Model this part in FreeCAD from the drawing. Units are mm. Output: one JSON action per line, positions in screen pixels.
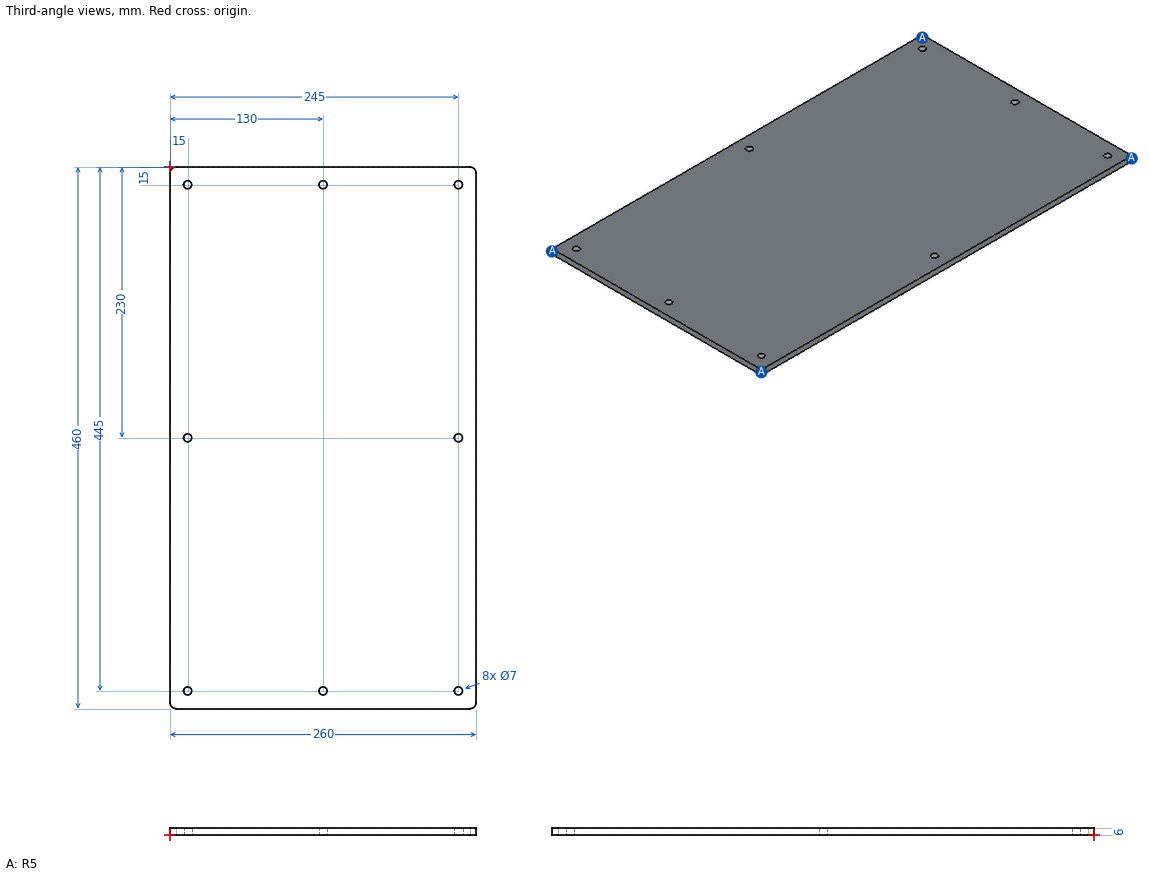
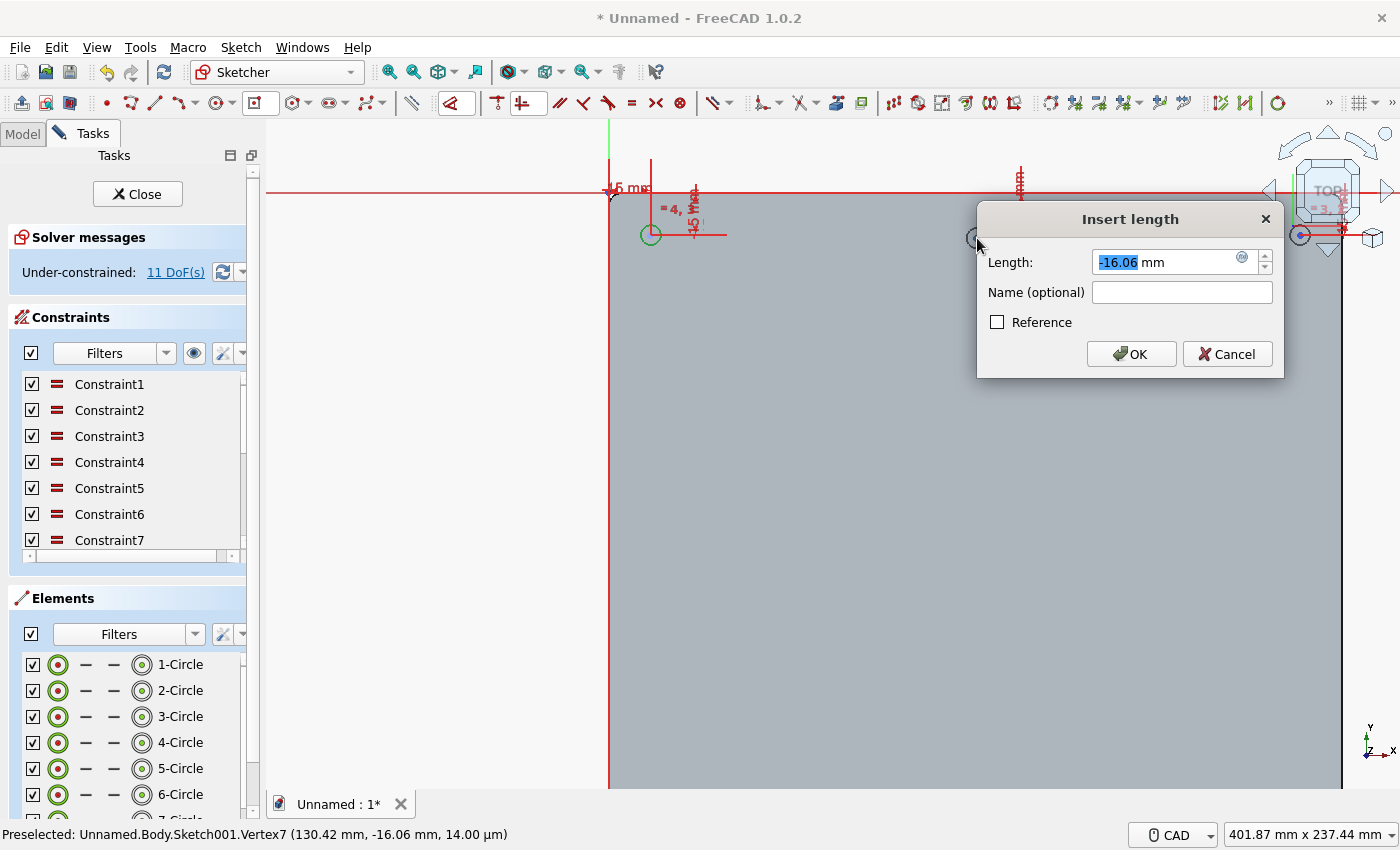
{"action": "type", "text": "-15"}
{"action": "key", "text": "Return"}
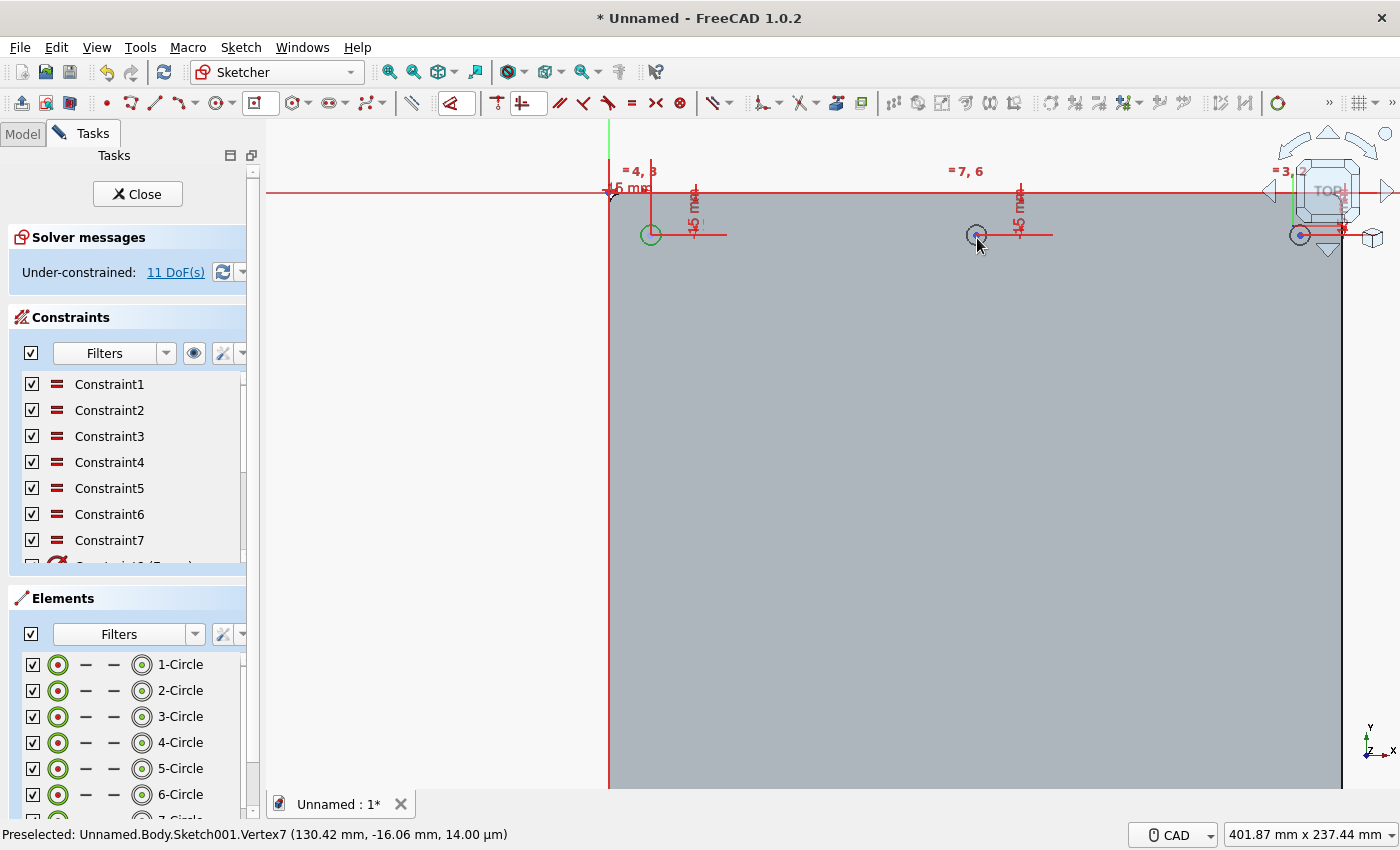
{"action": "scroll", "coordinate": [651, 238], "scroll_direction": "down", "scroll_amount": 5}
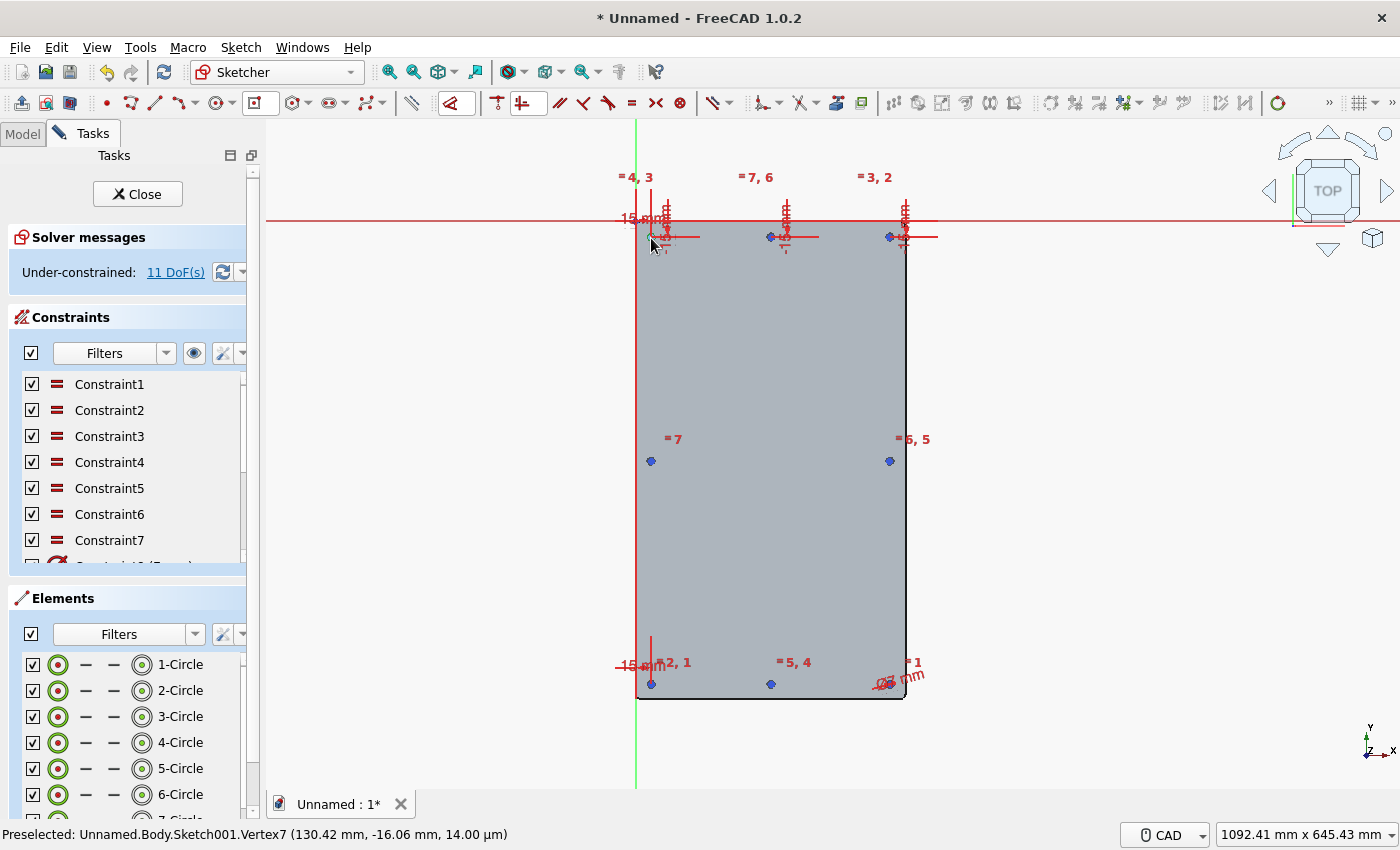
{"action": "scroll", "coordinate": [651, 461], "scroll_direction": "up", "scroll_amount": 5}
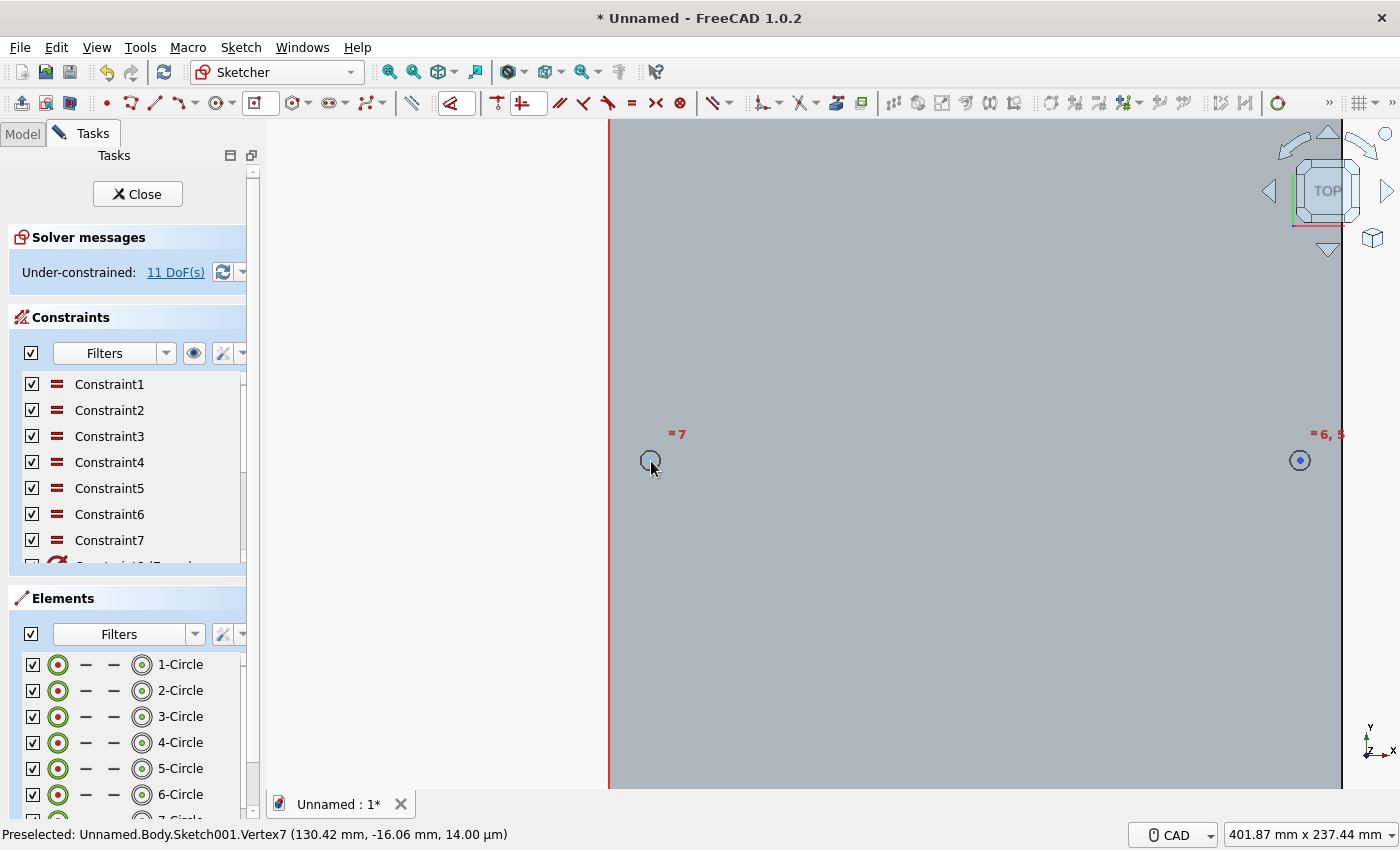
{"action": "left_click", "coordinate": [650, 461]}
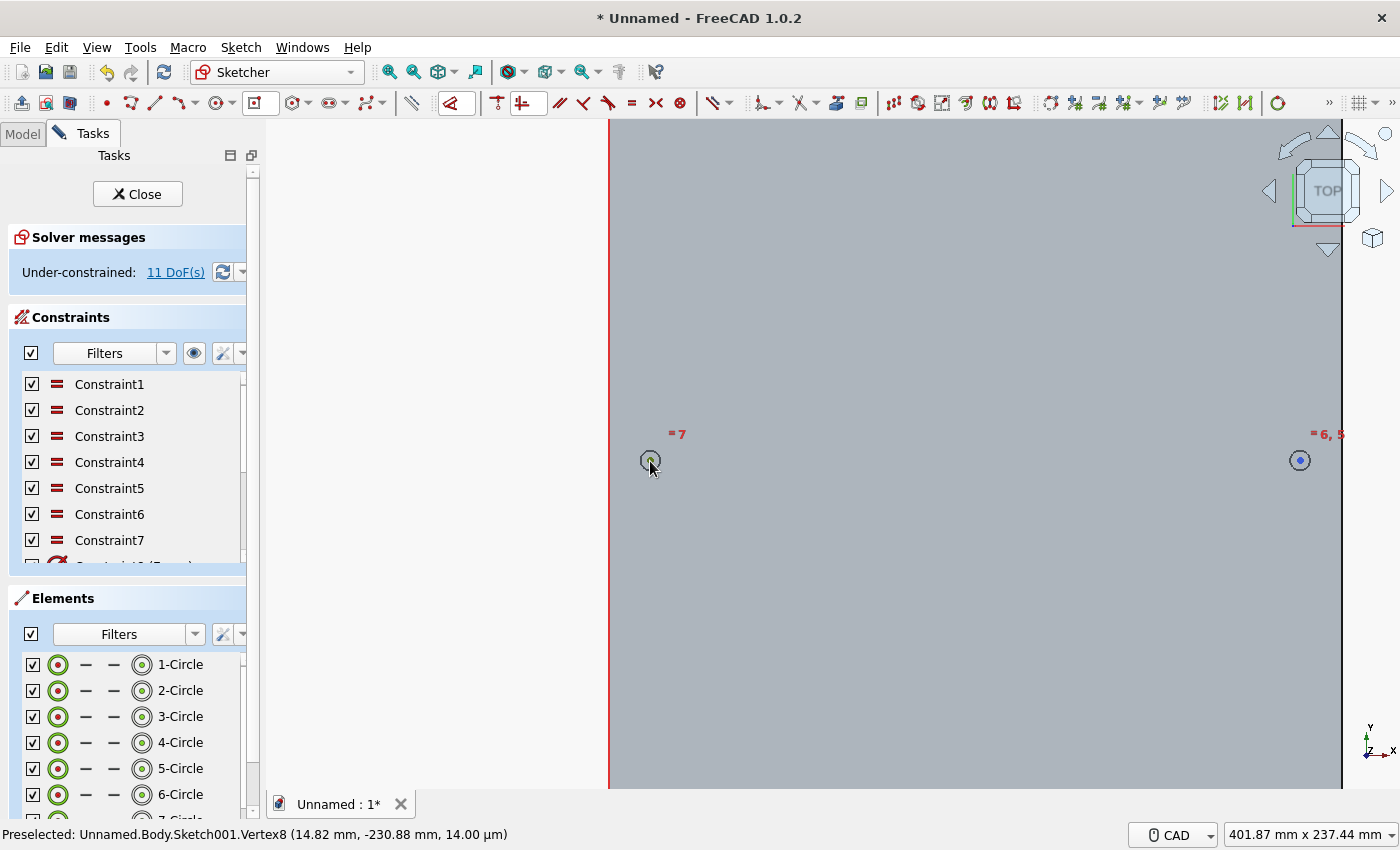
{"action": "key", "text": "l"}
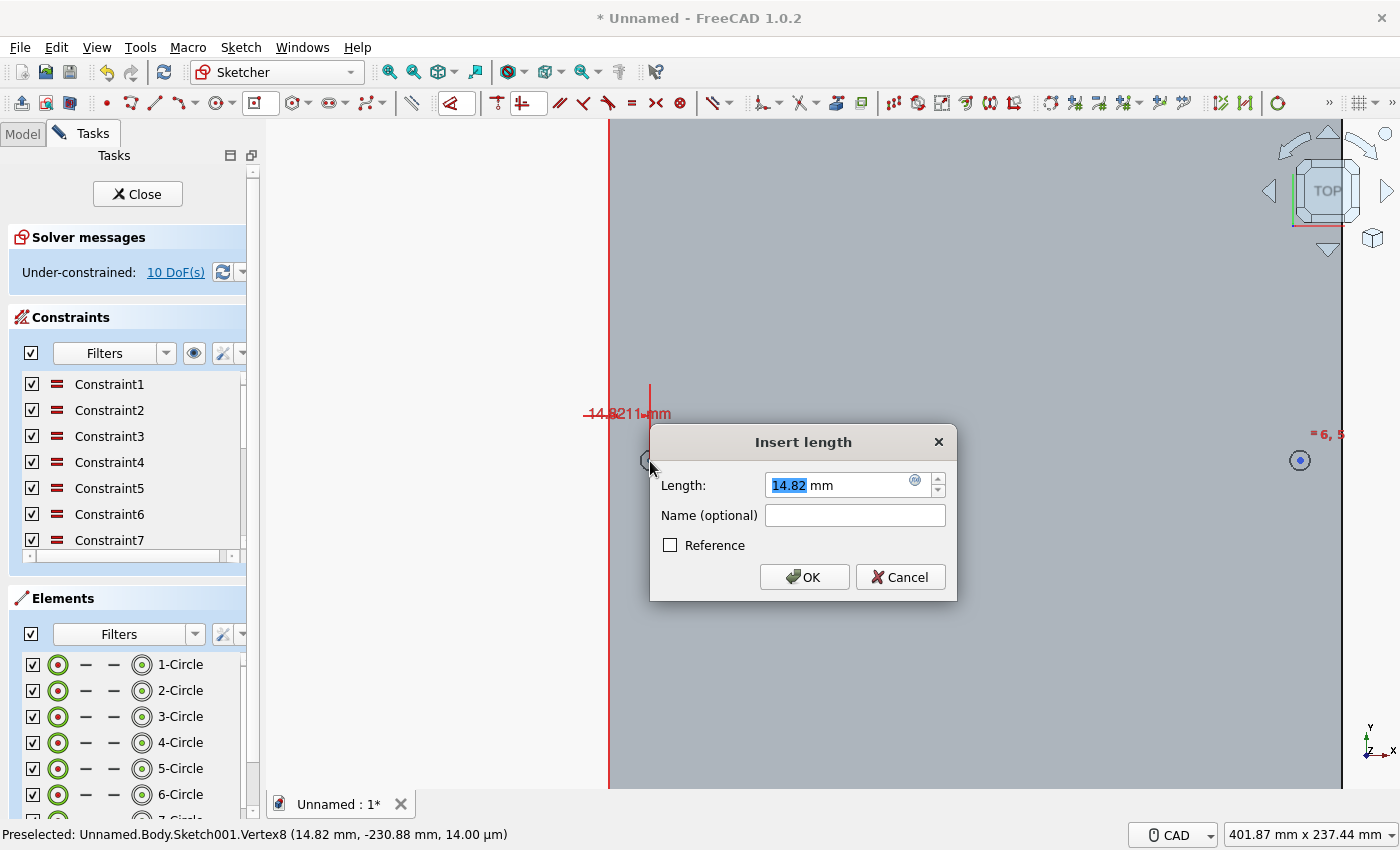
{"action": "type", "text": "15"}
{"action": "key", "text": "Return"}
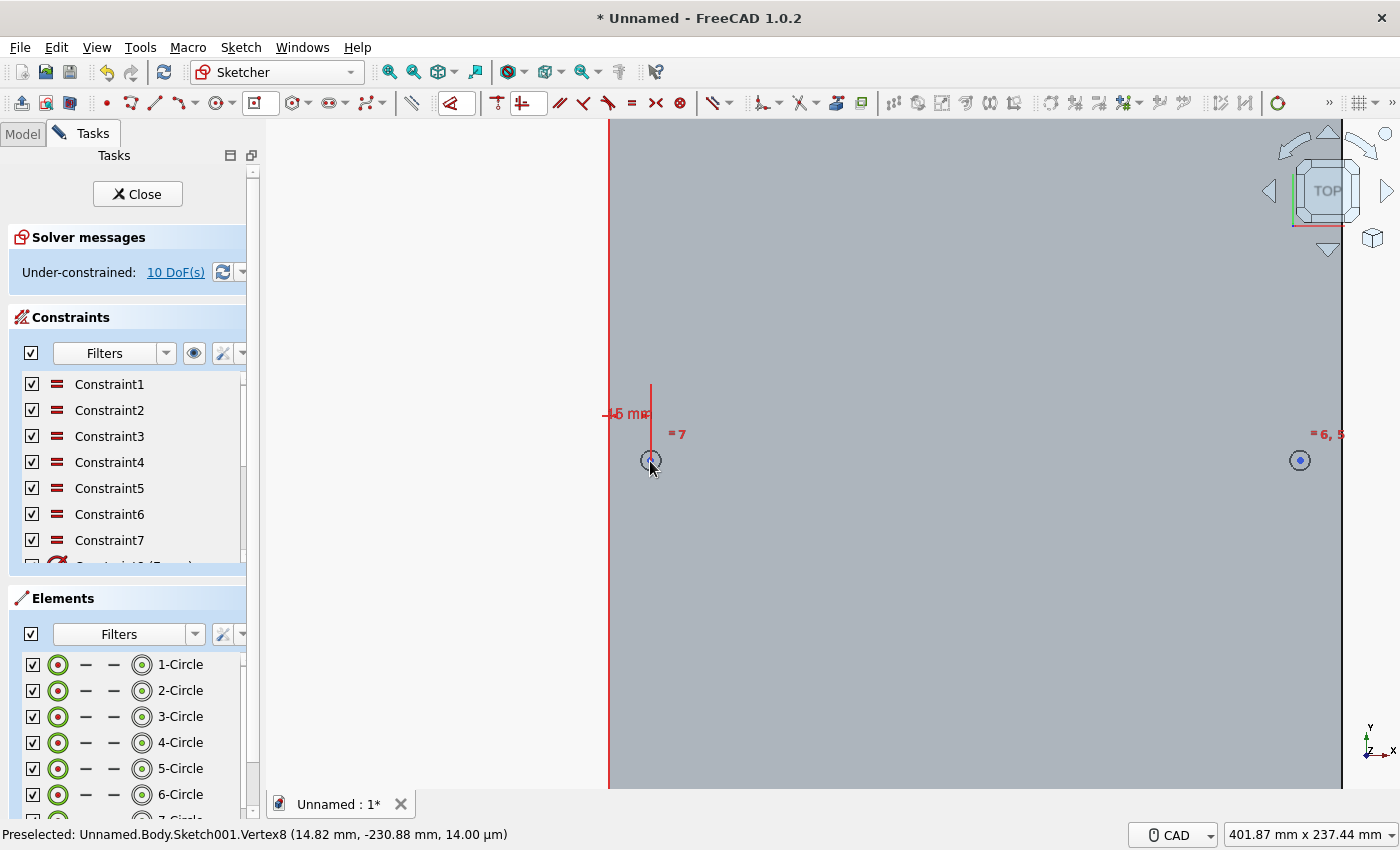
{"action": "scroll", "coordinate": [651, 461], "scroll_direction": "down", "scroll_amount": 5}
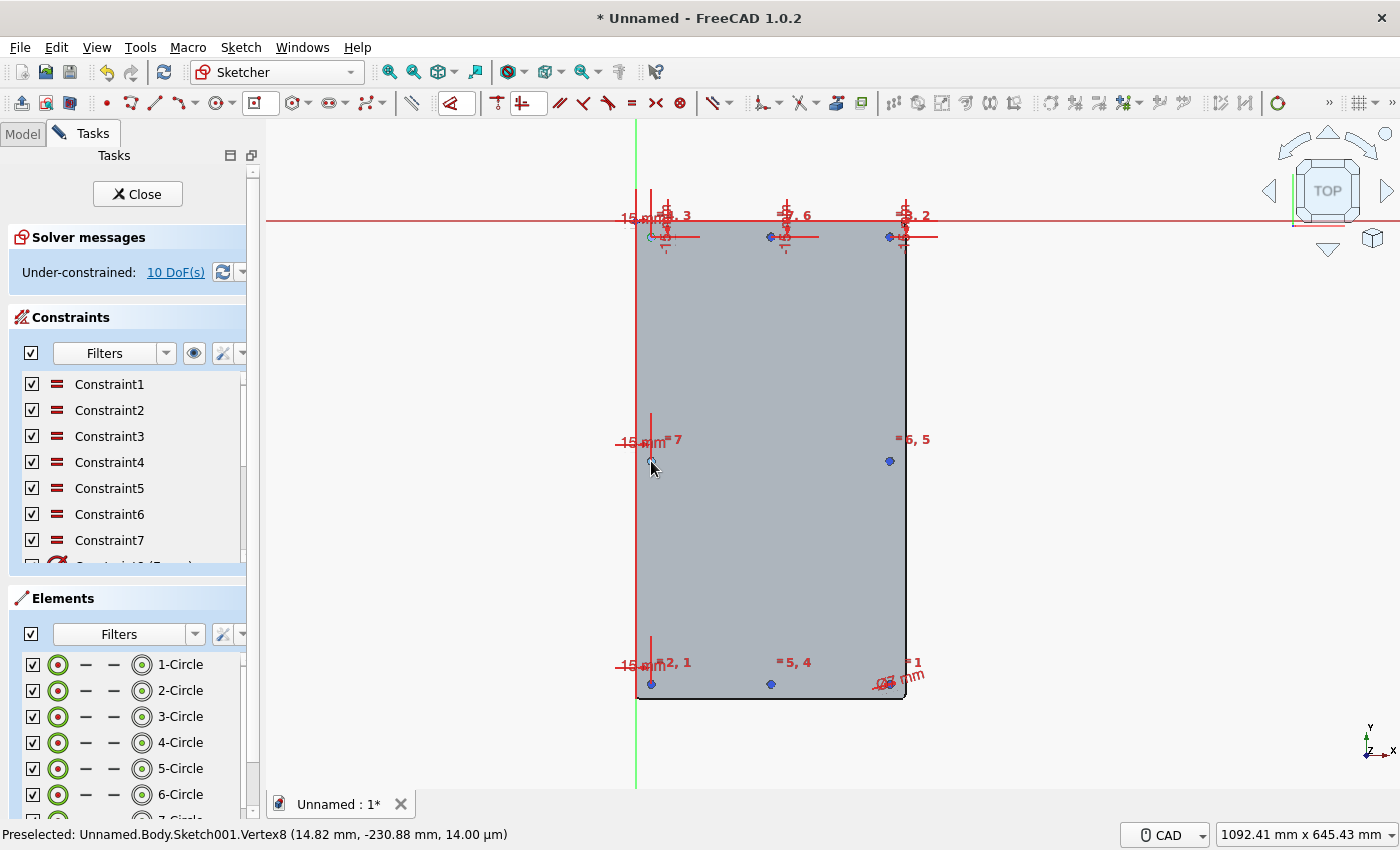
{"action": "left_click", "coordinate": [890, 684]}